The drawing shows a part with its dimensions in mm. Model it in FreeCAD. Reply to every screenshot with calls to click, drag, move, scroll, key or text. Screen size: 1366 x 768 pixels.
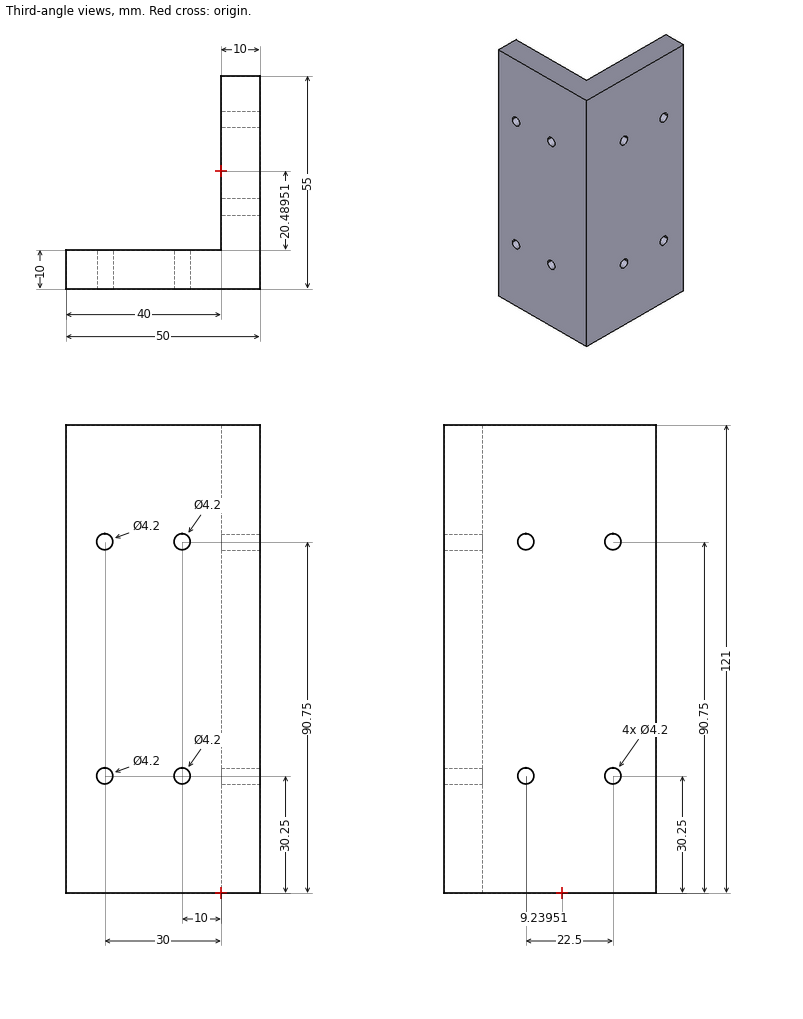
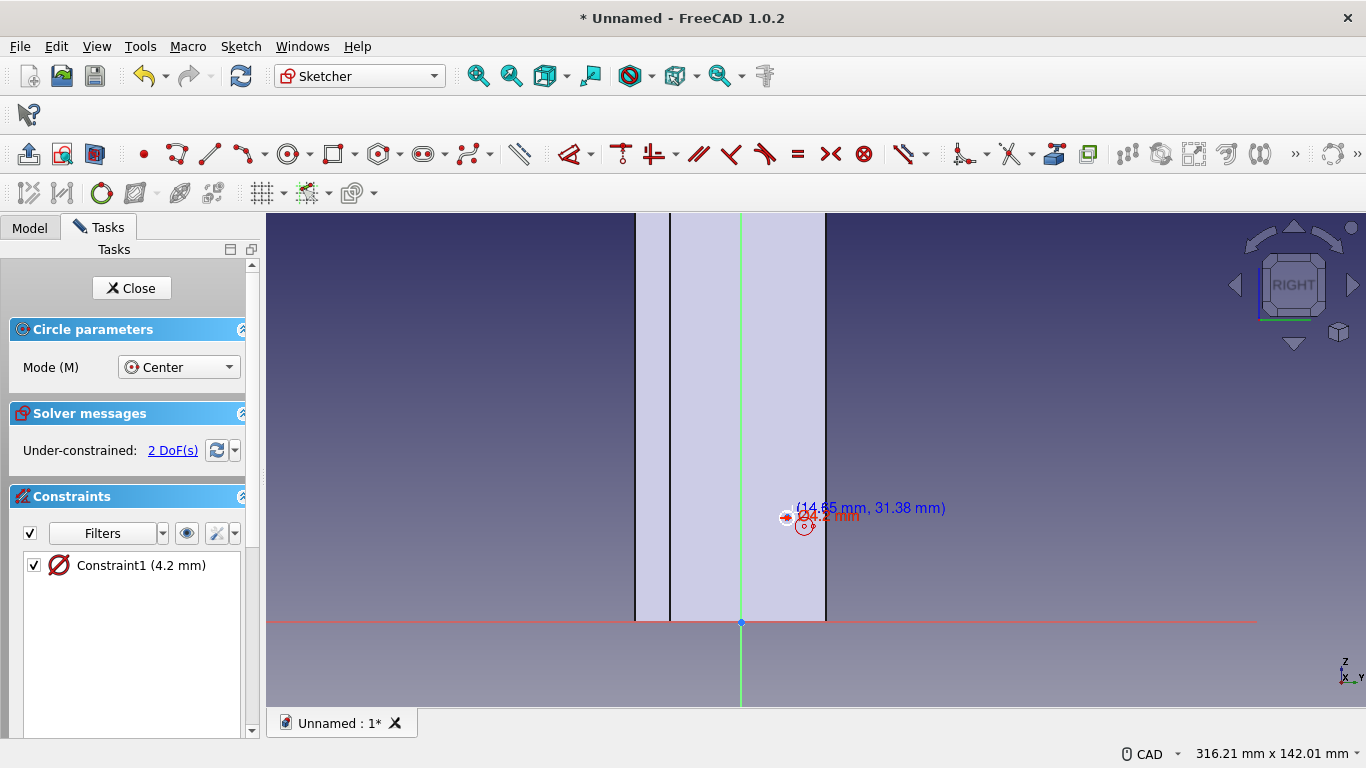
scroll(709, 517, up, 6)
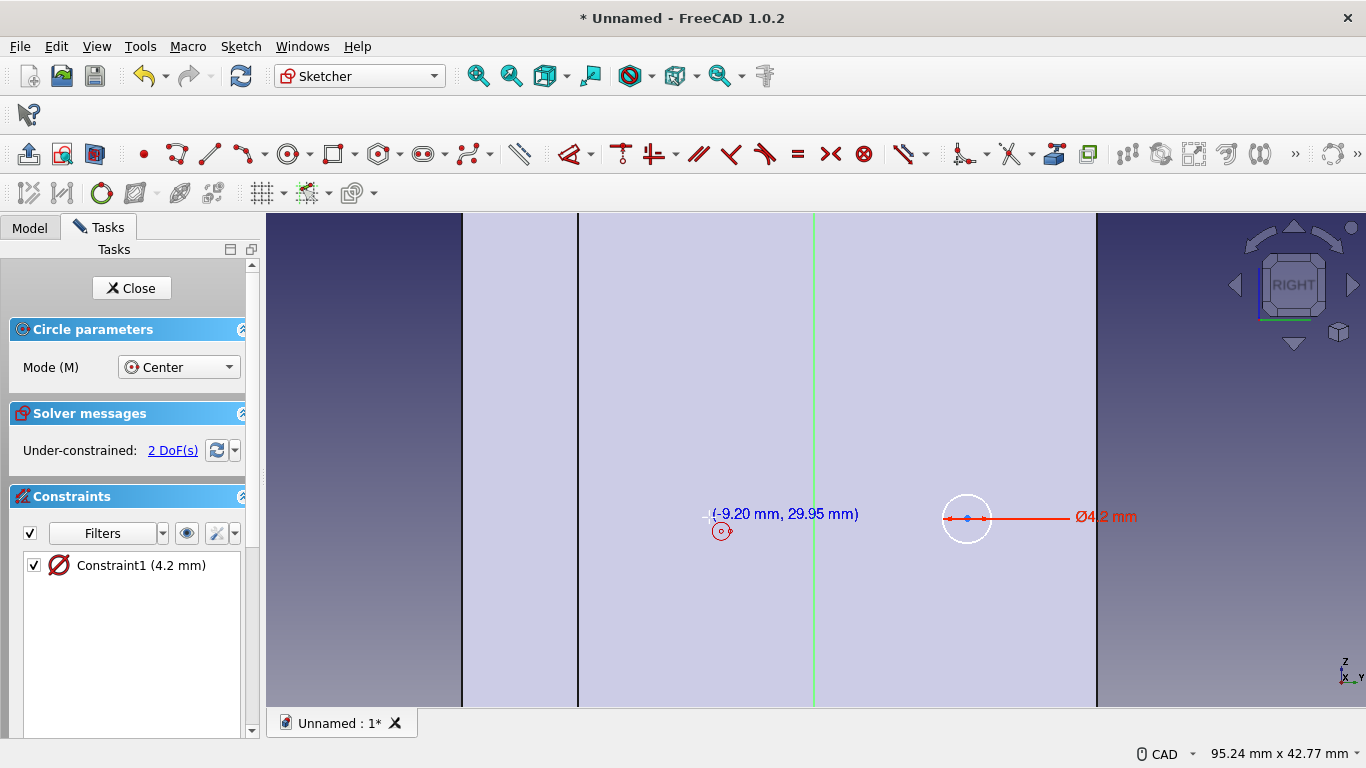
scroll(709, 517, down, 6)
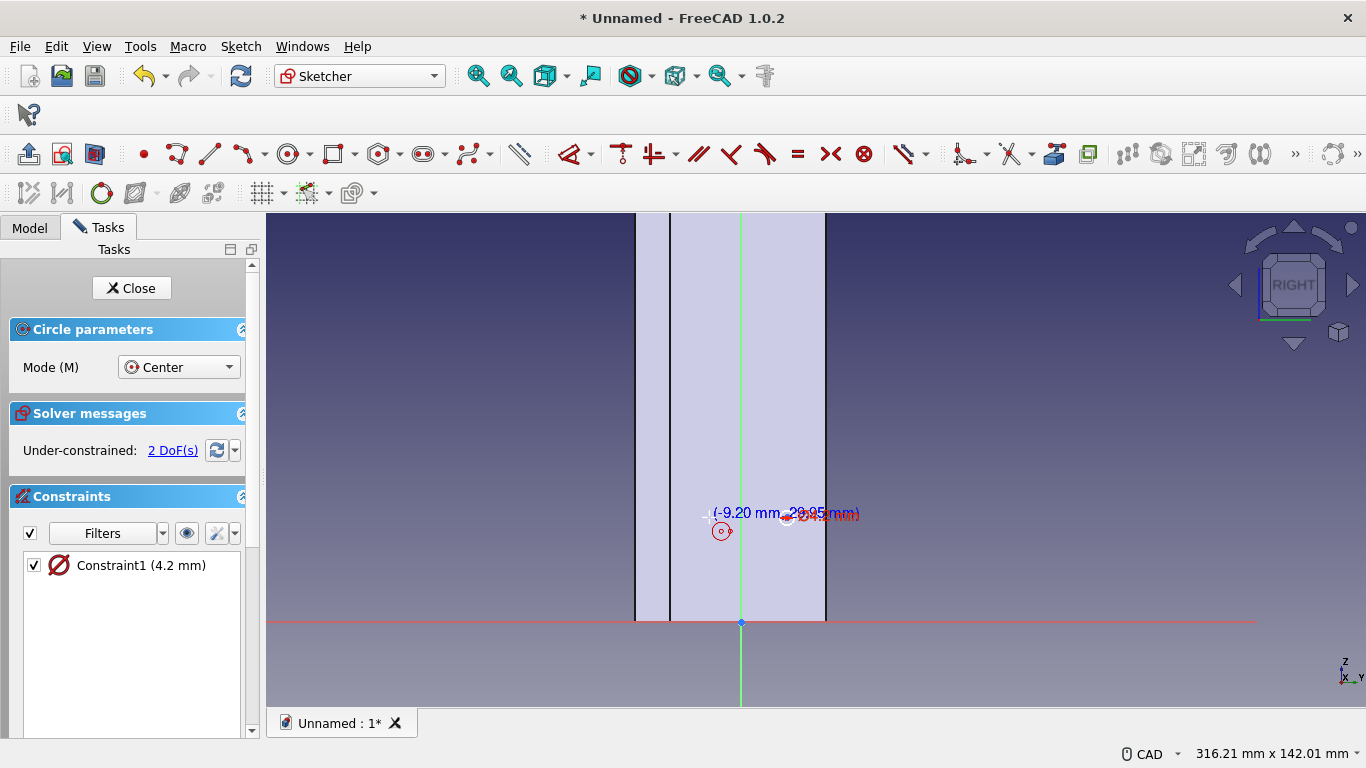
click(709, 517)
move(714, 512)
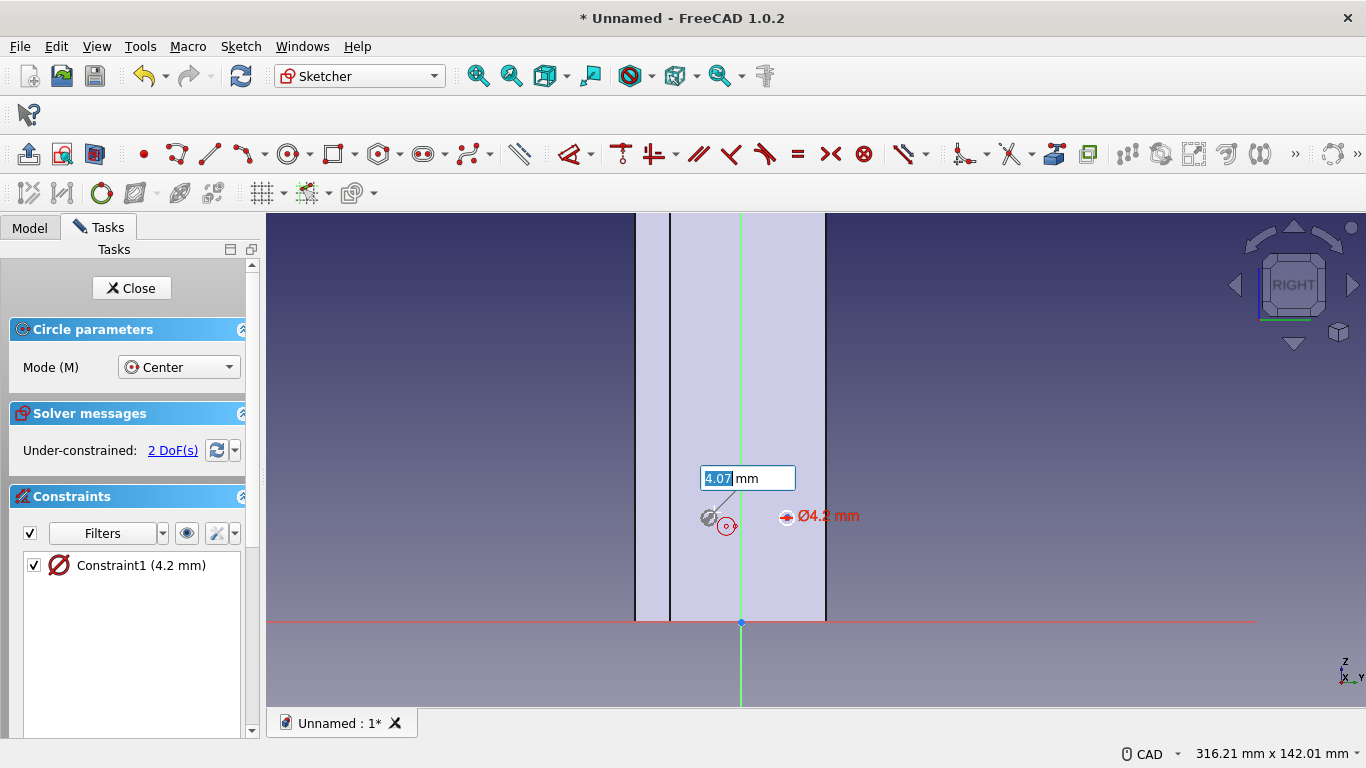
text(4.2)
key(Return)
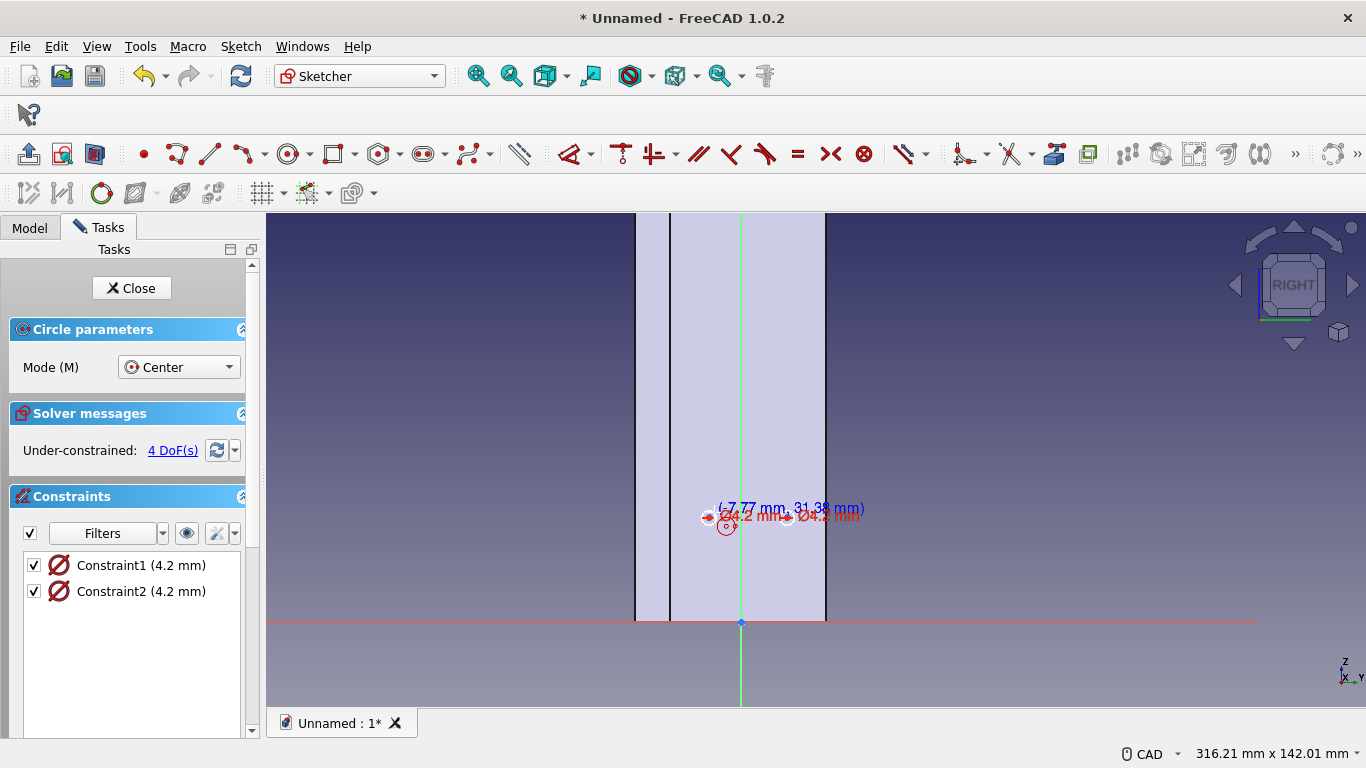
scroll(787, 306, up, 6)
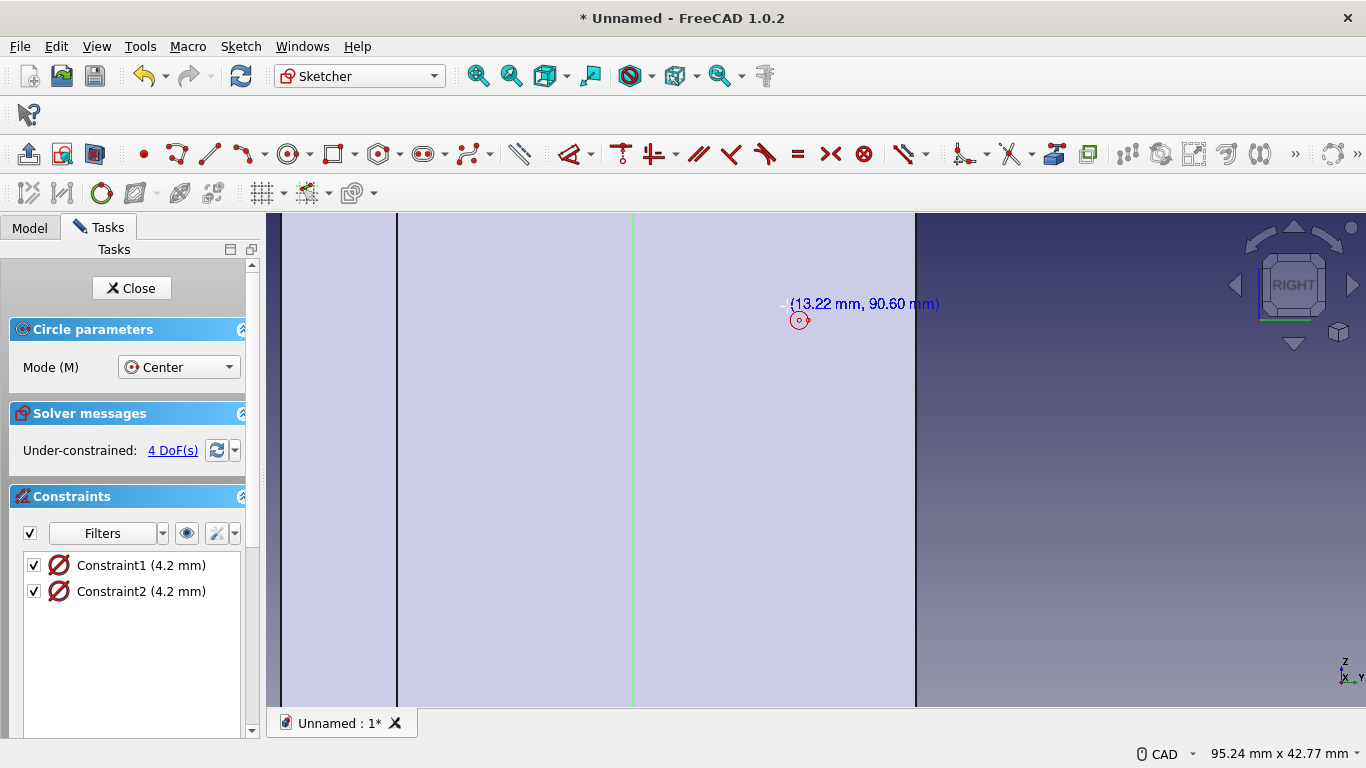
scroll(787, 305, down, 6)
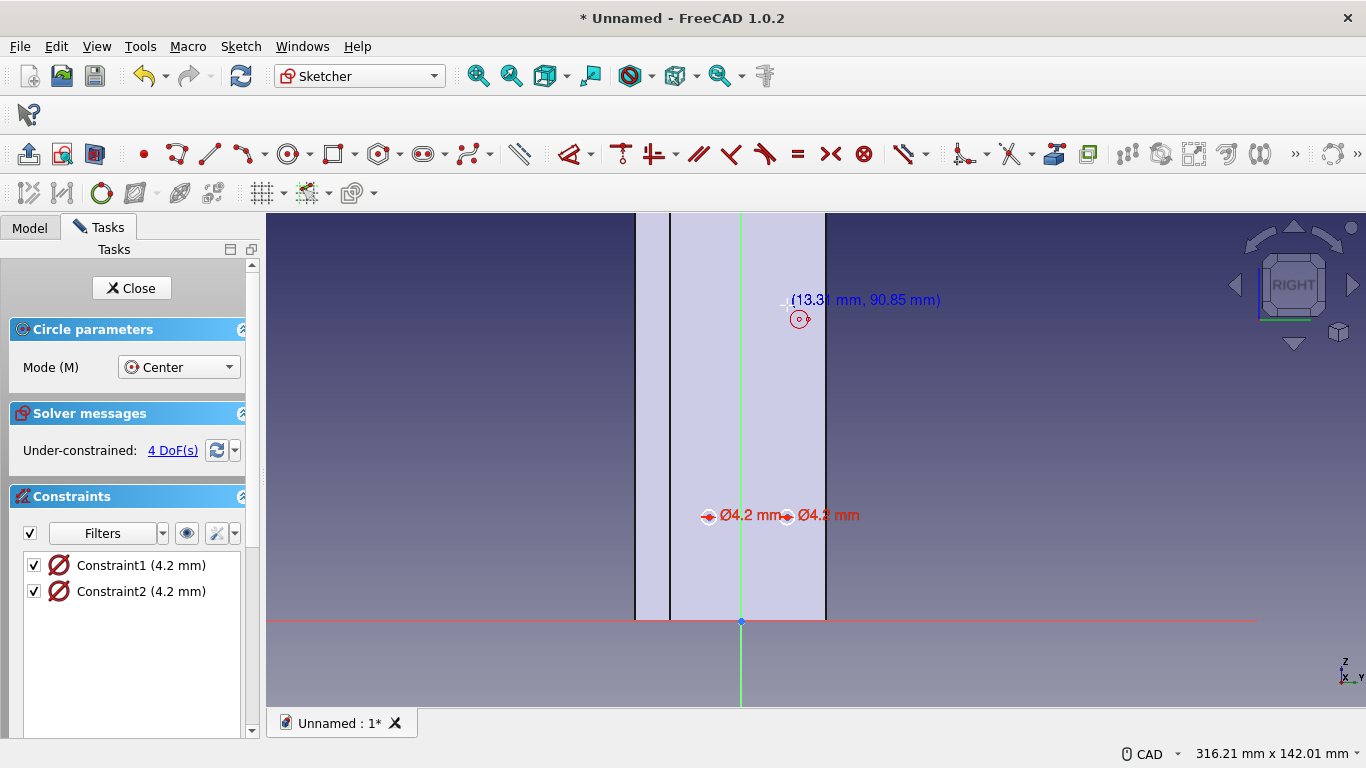
click(787, 306)
move(792, 301)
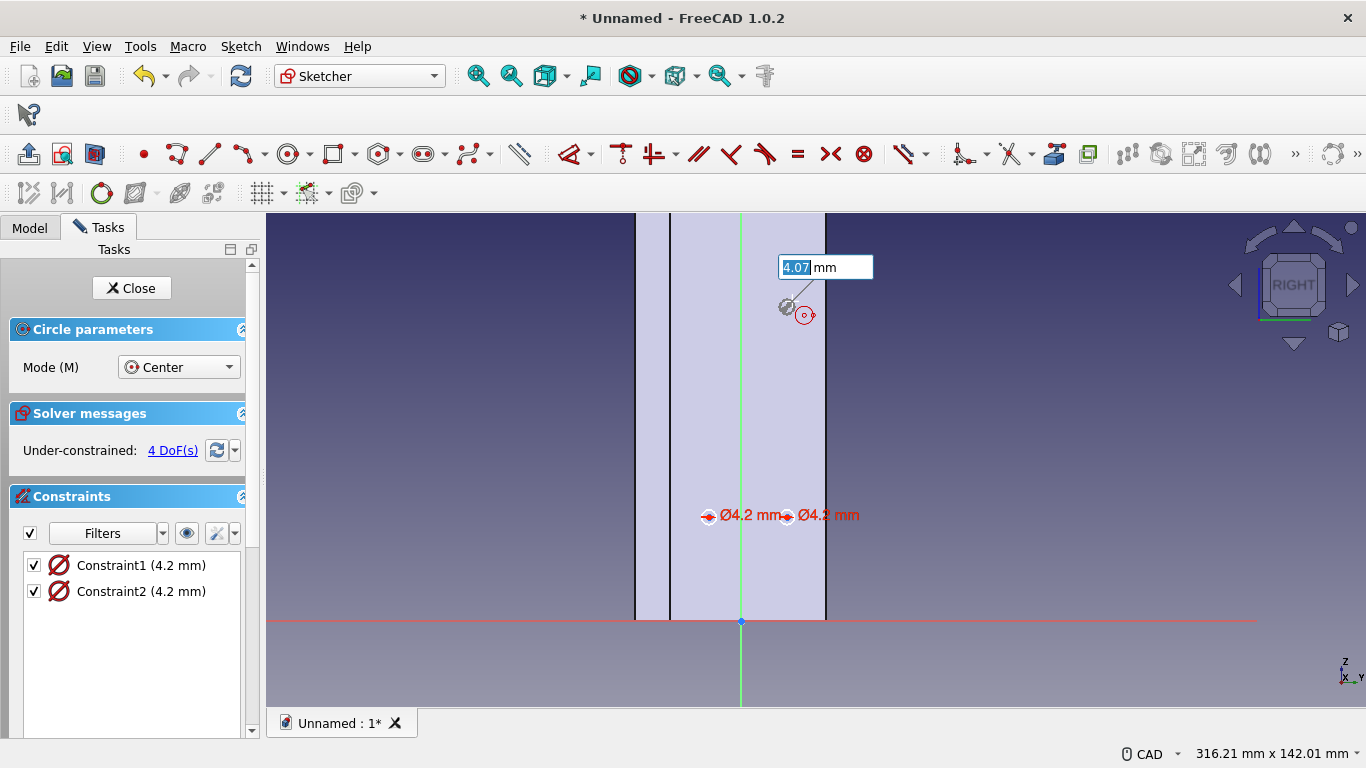
text(4.2)
key(Return)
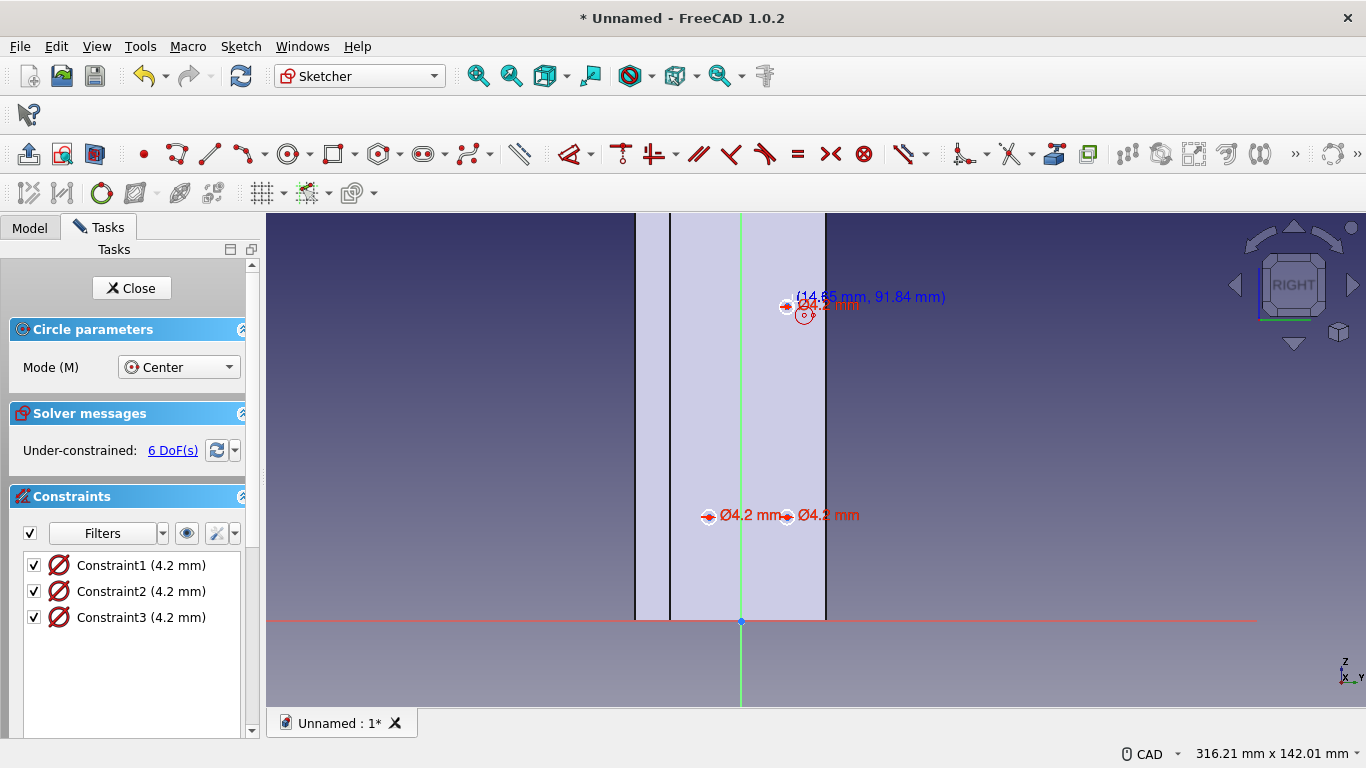
scroll(709, 306, up, 6)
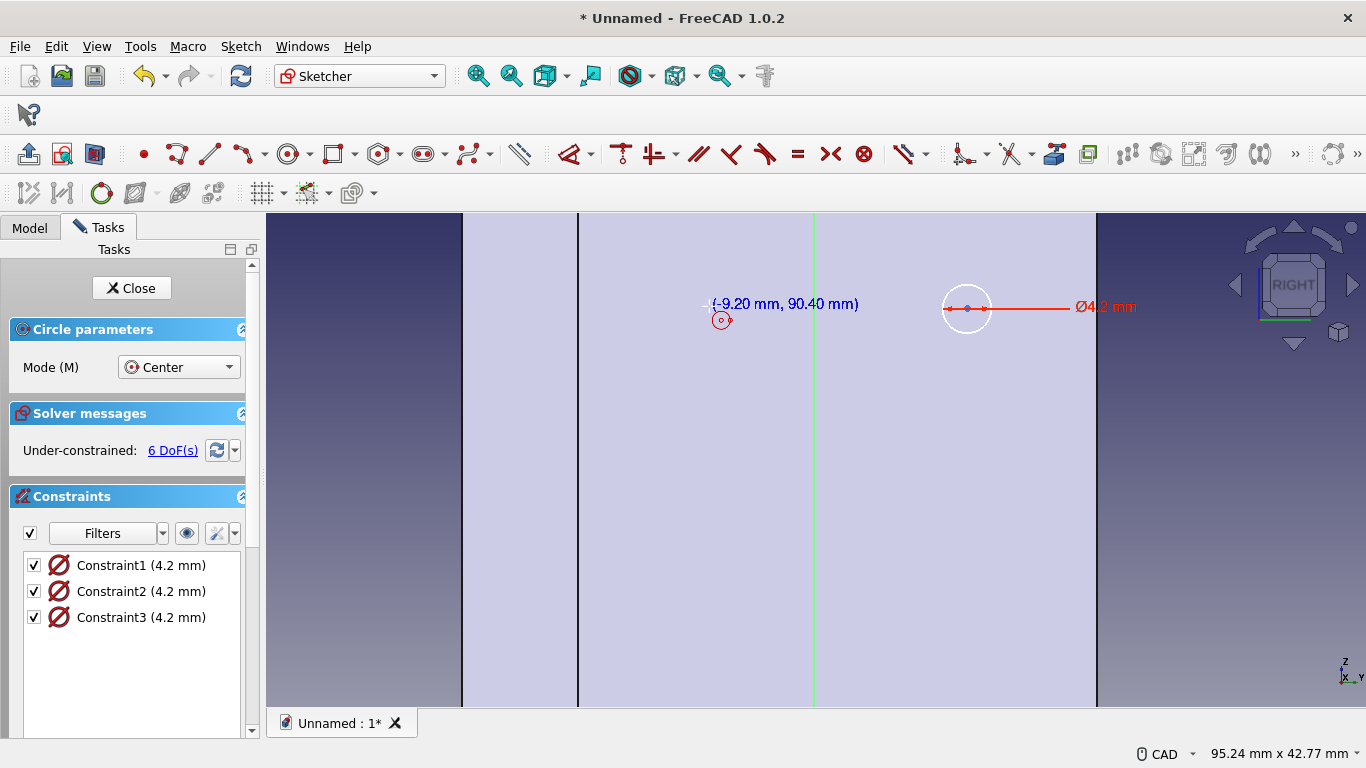
scroll(709, 306, down, 6)